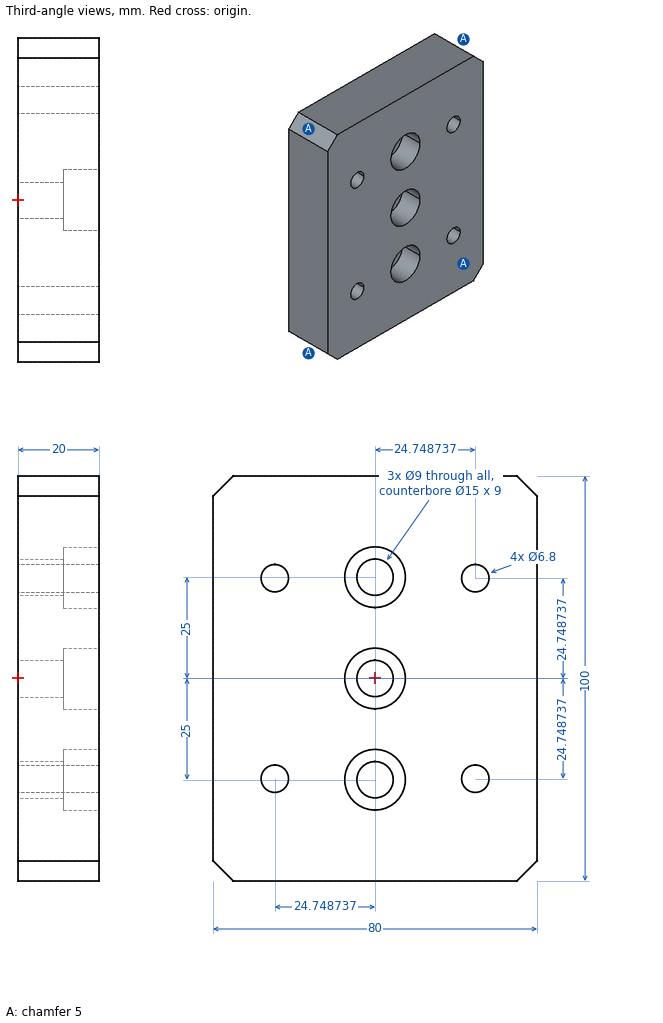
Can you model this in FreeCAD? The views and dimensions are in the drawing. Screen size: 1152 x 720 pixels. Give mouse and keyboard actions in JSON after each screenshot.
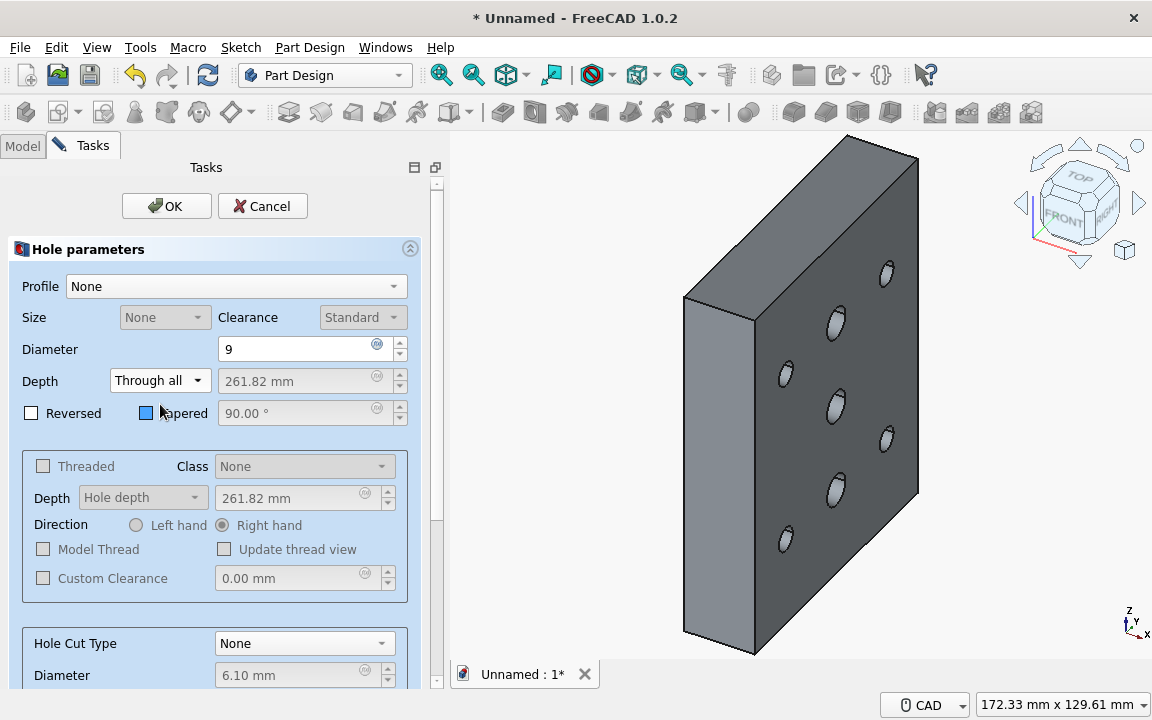
{"action": "left_click", "coordinate": [306, 644]}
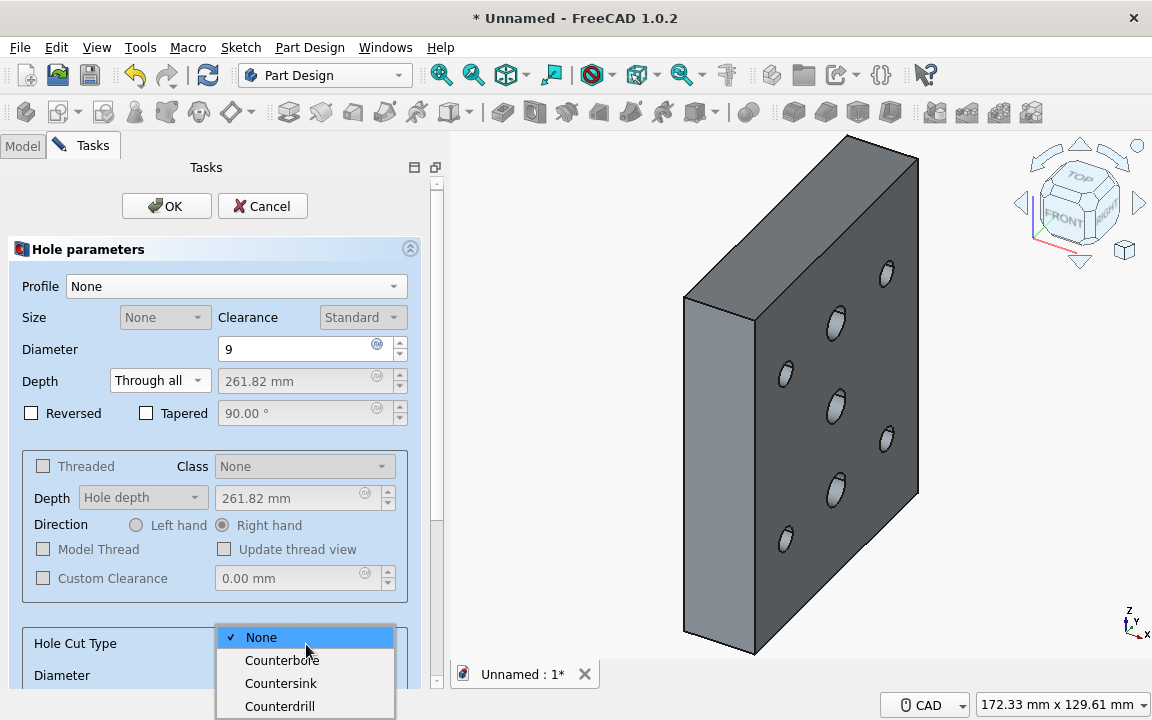
{"action": "left_click", "coordinate": [304, 660]}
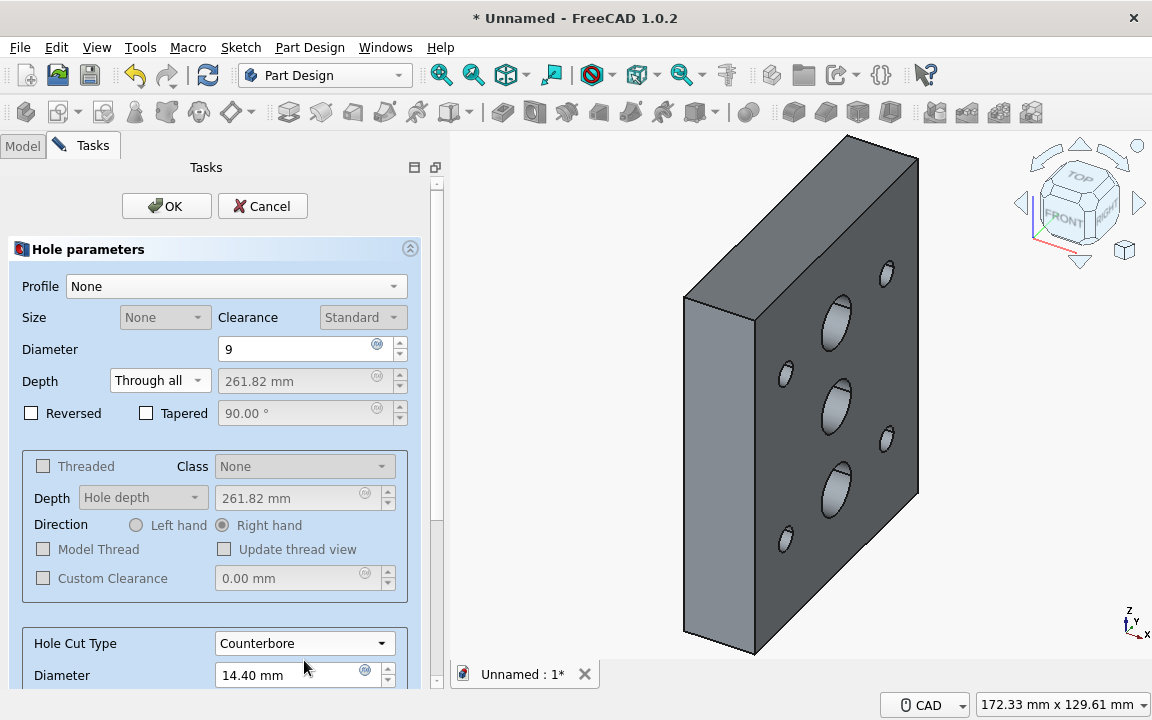
{"action": "triple_click", "coordinate": [298, 675]}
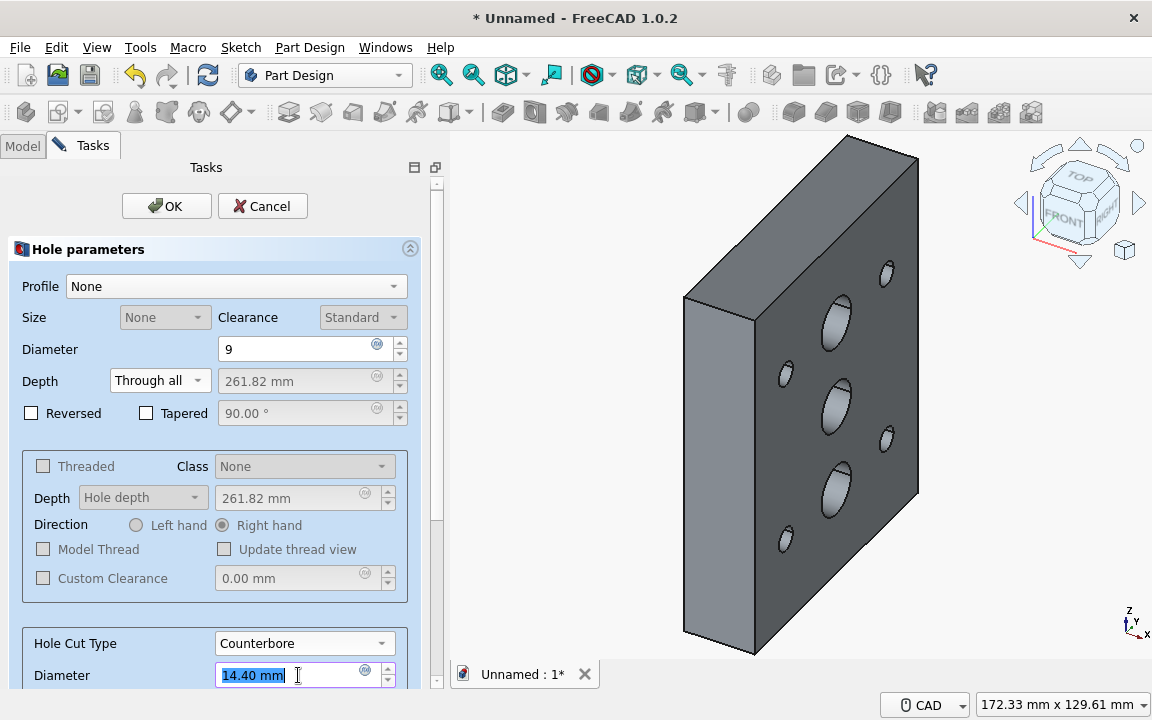
{"action": "type", "text": "15"}
{"action": "key", "text": "Tab"}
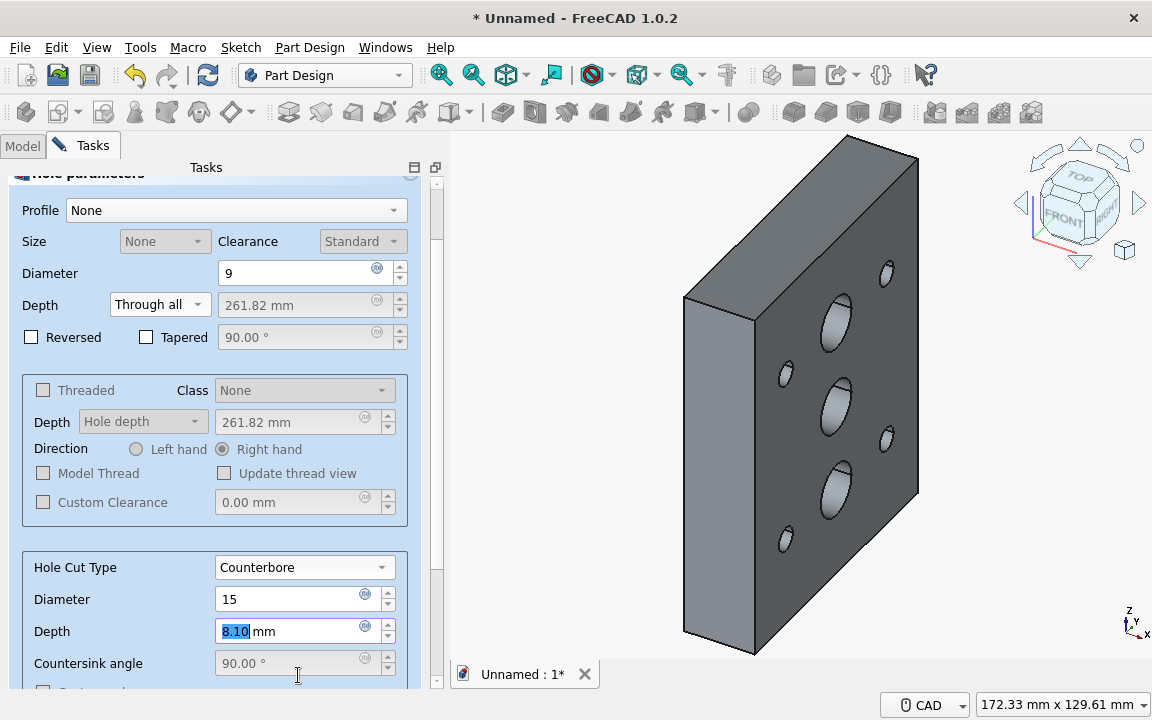
{"action": "type", "text": "9"}
{"action": "key", "text": "Tab"}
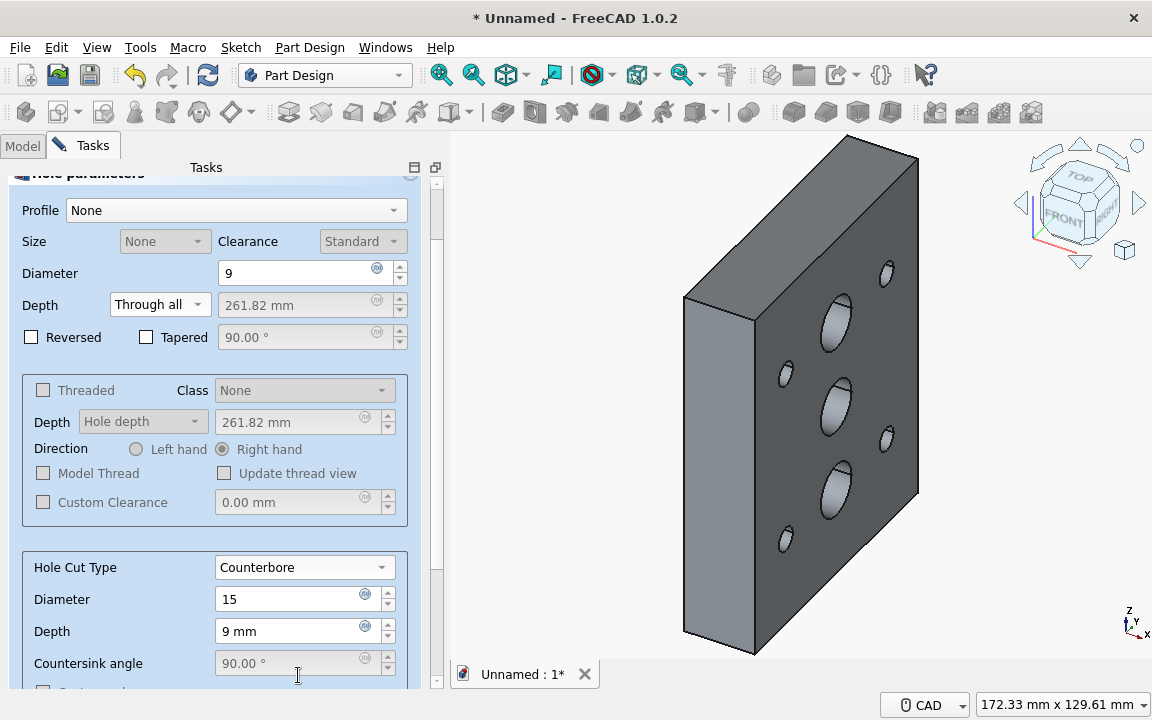
{"action": "scroll", "coordinate": [437, 432], "scroll_direction": "up", "scroll_amount": 3}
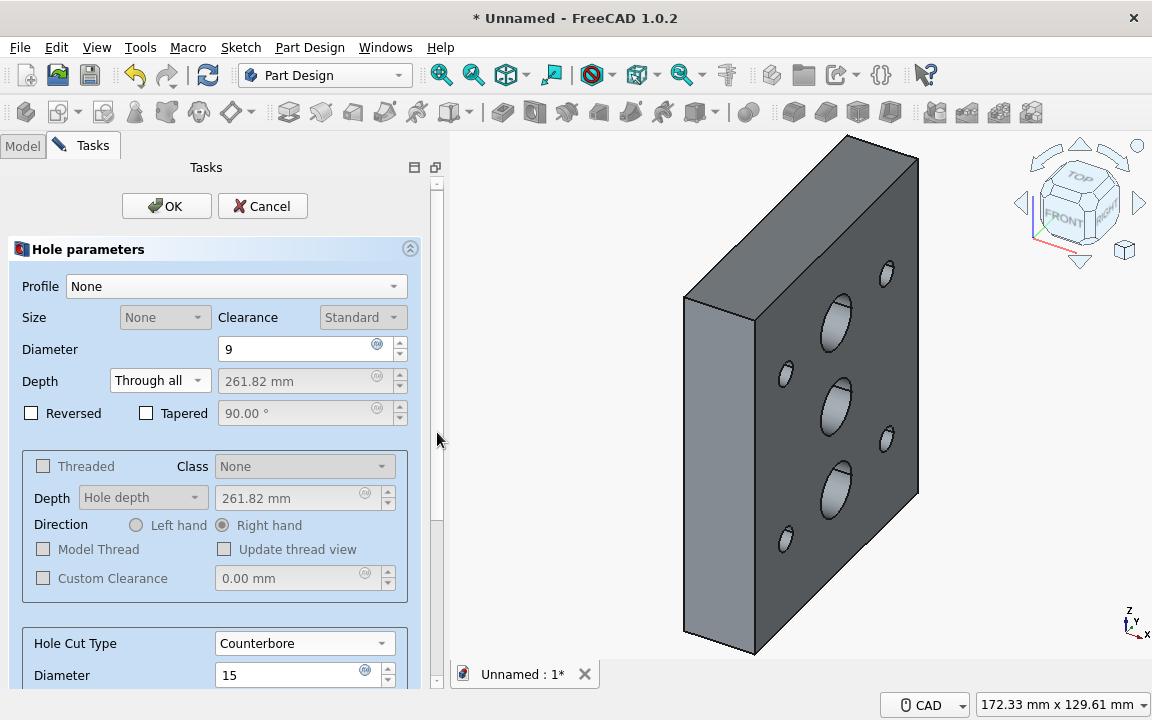
{"action": "left_click", "coordinate": [167, 206]}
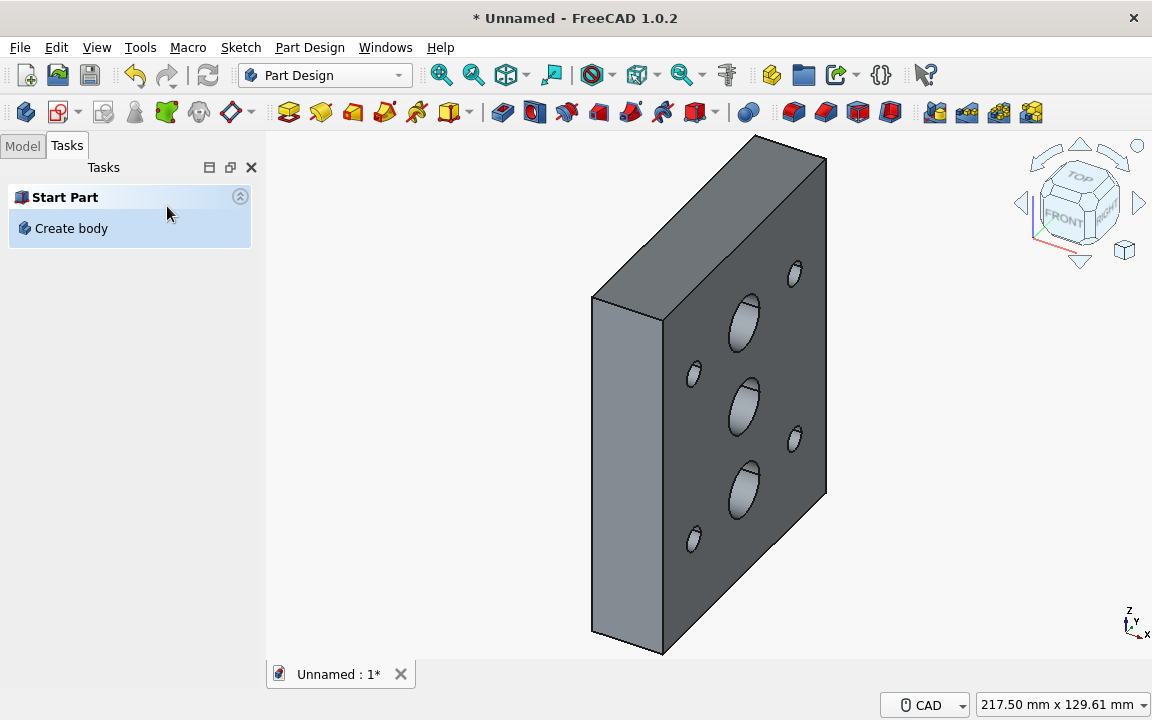
{"action": "left_click", "coordinate": [628, 308]}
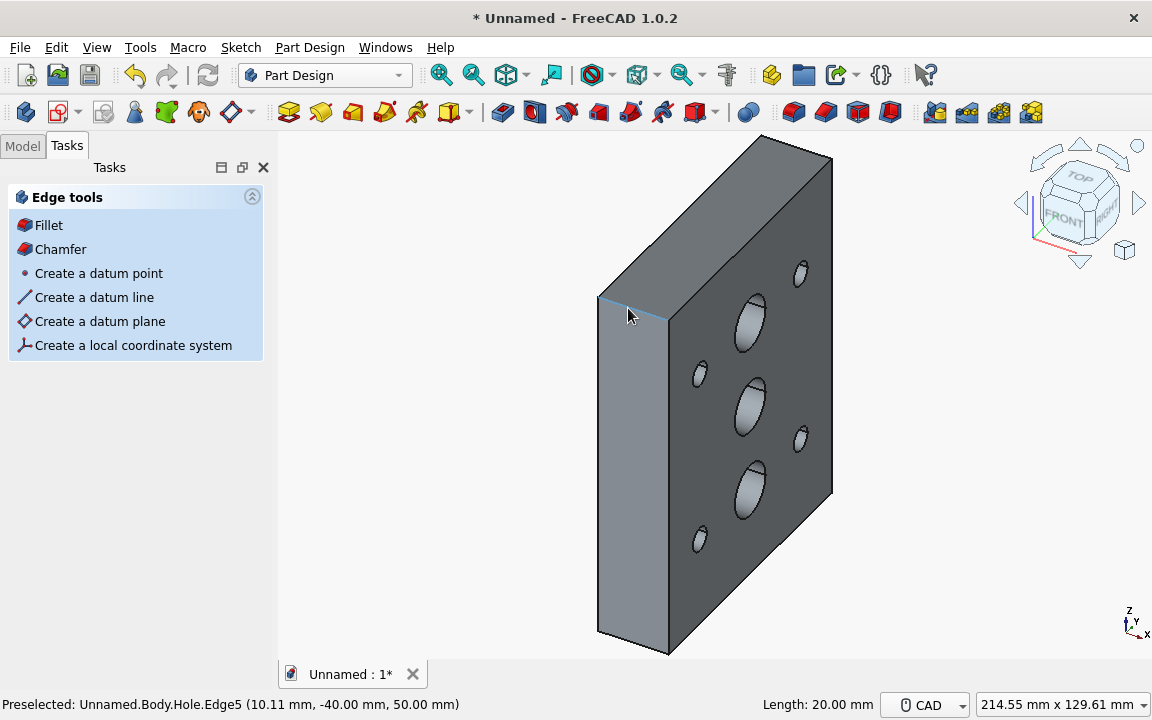
{"action": "key", "text": "0"}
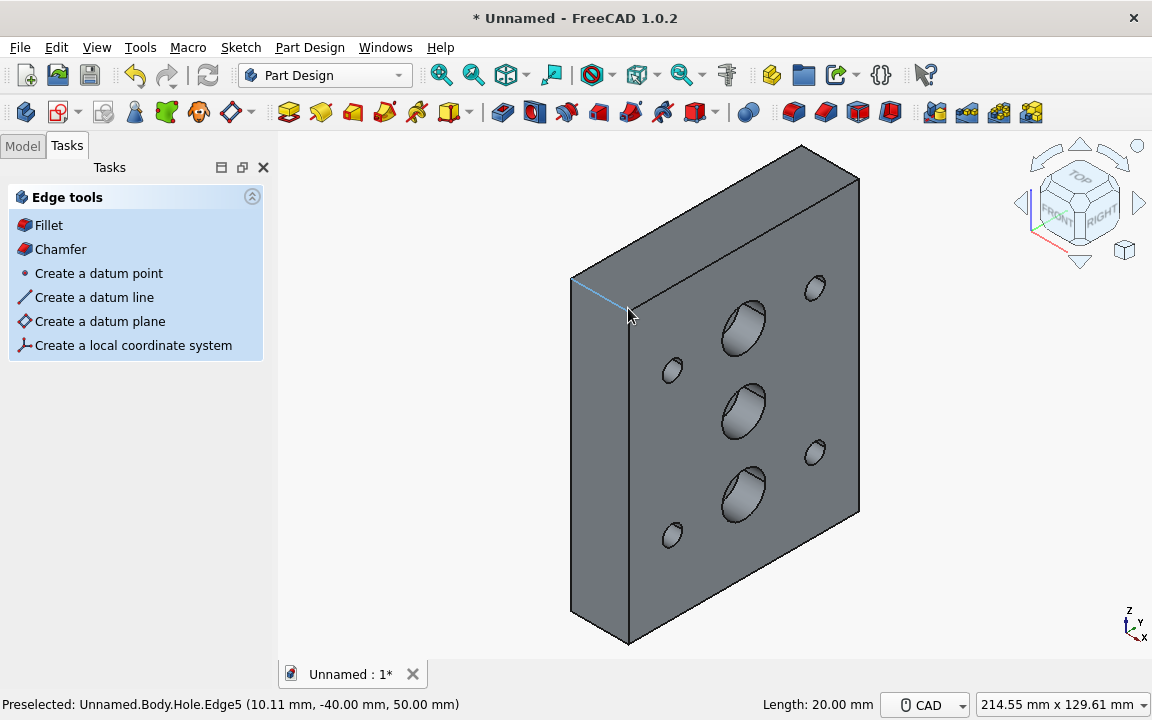
{"action": "key", "text": "2"}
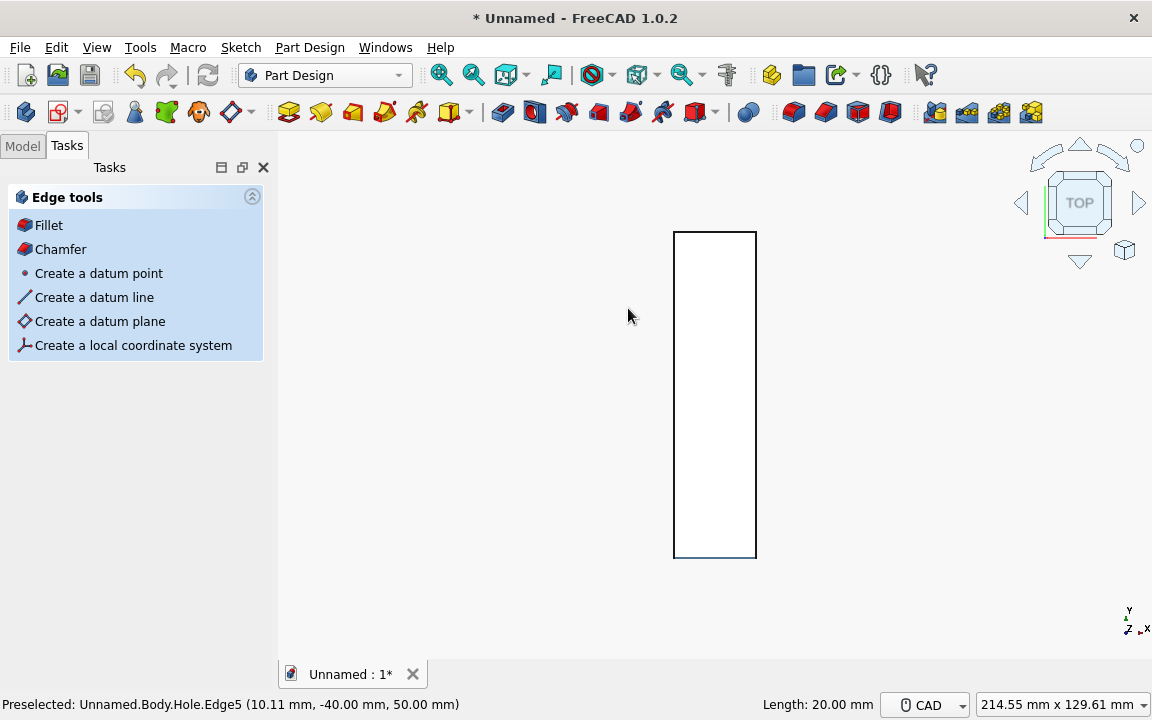
{"action": "left_click", "coordinate": [715, 231], "text": "ctrl"}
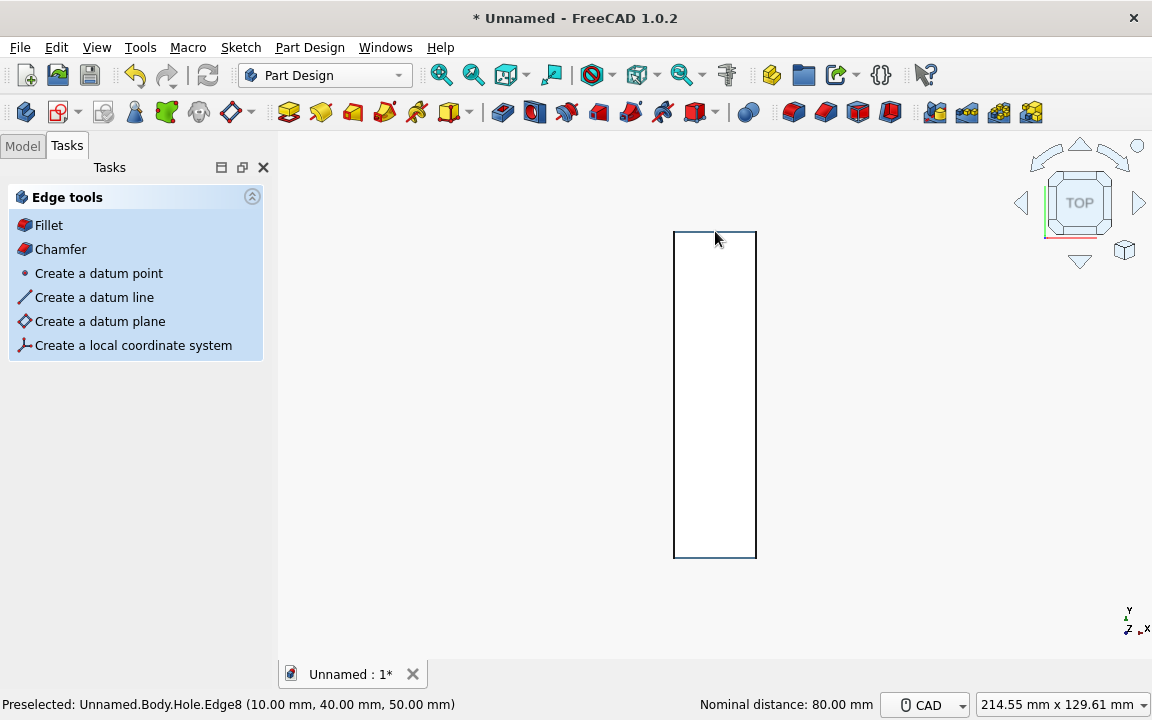
{"action": "key", "text": "1"}